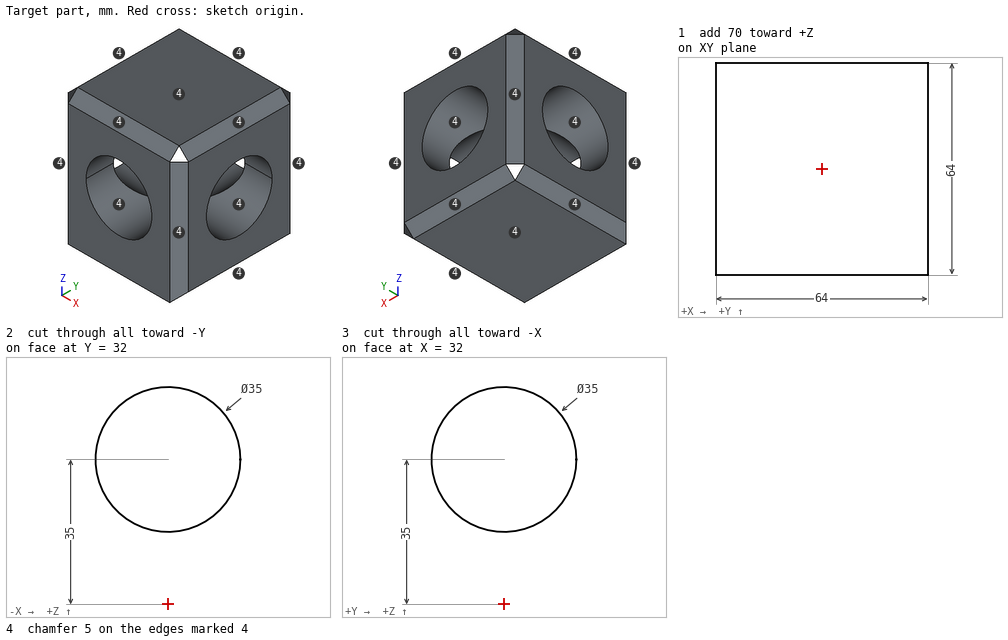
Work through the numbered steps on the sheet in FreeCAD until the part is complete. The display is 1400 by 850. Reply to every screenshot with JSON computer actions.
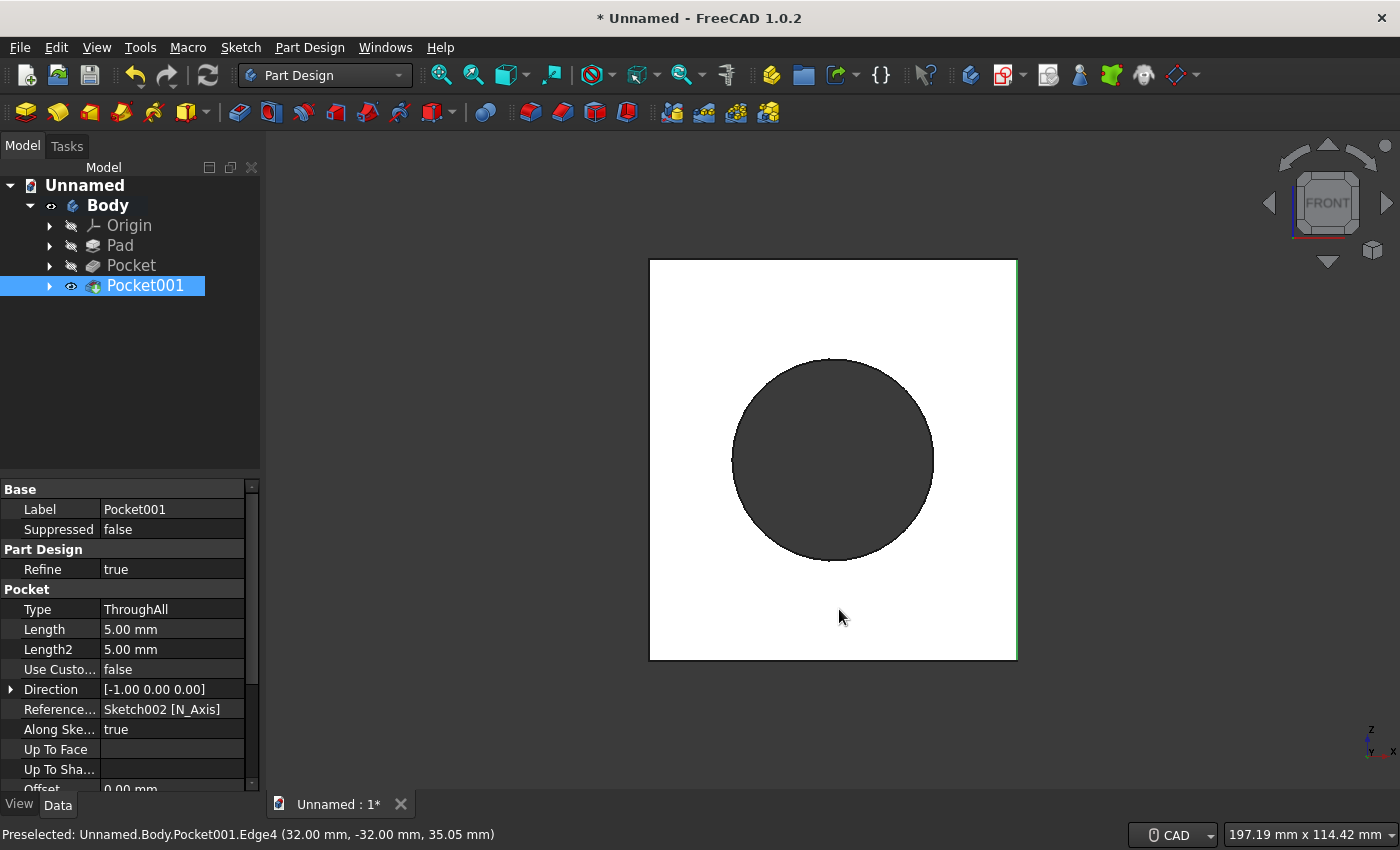
{"action": "left_click", "coordinate": [649, 459], "text": "ctrl"}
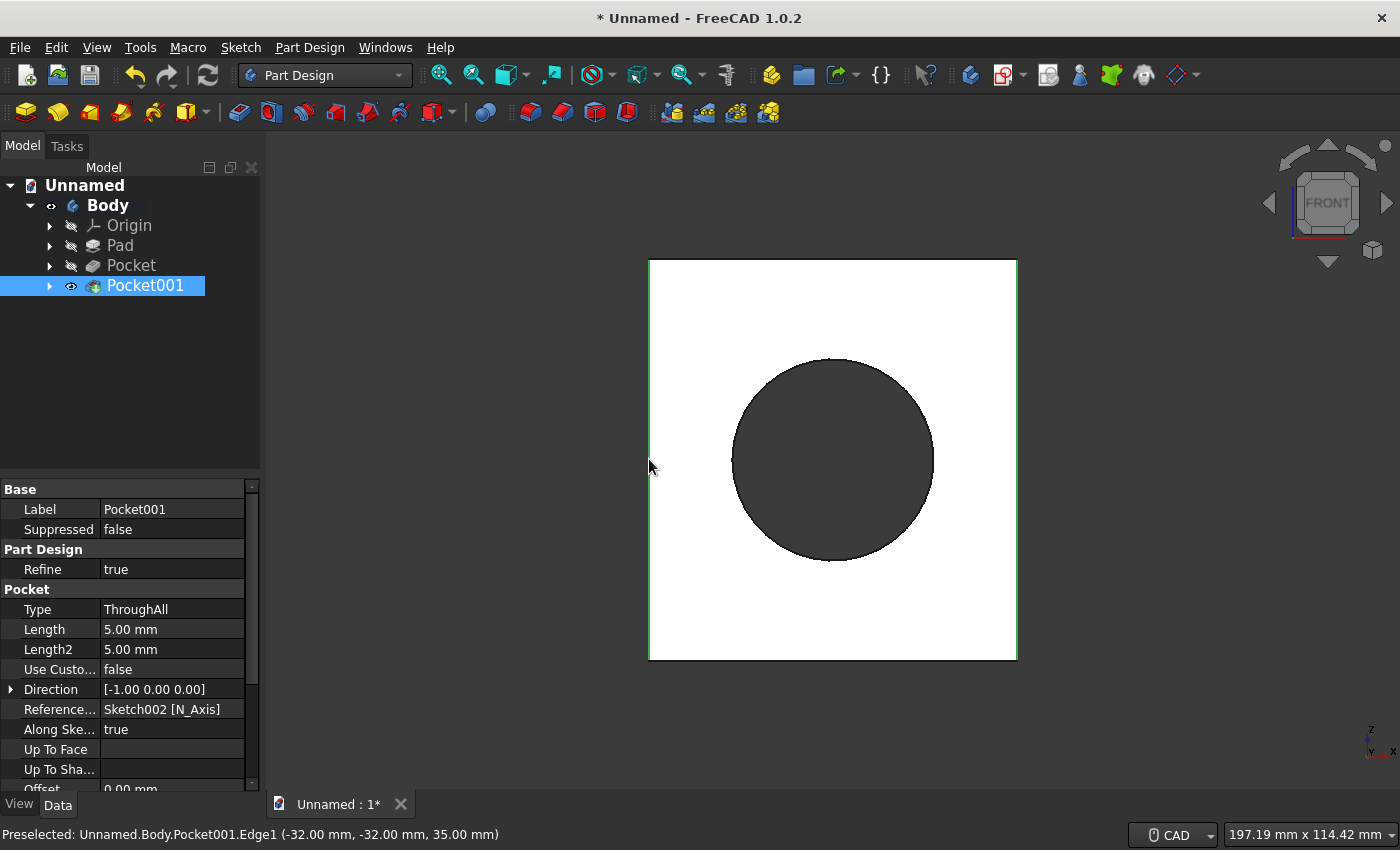
{"action": "key", "text": "3"}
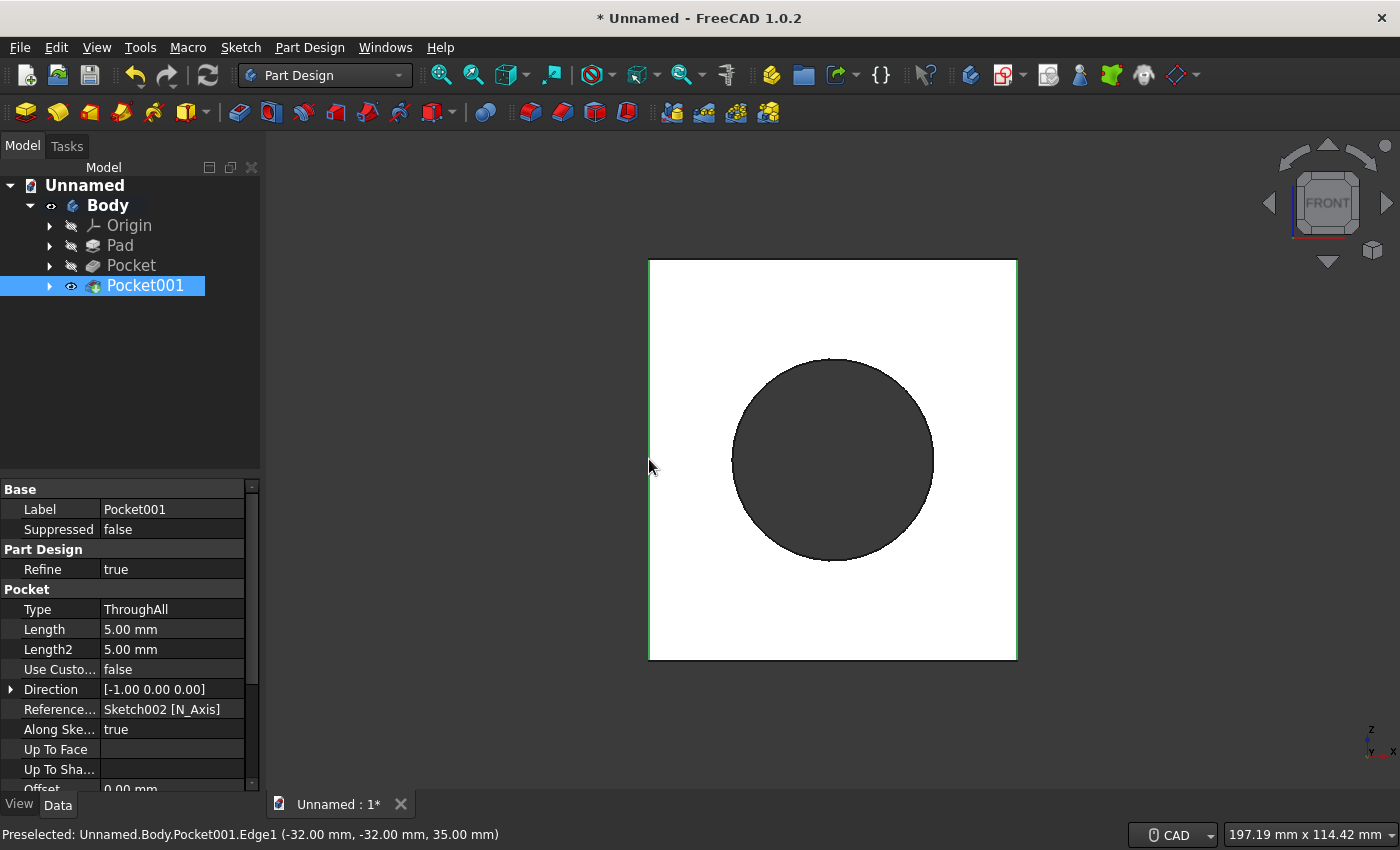
{"action": "left_click", "coordinate": [833, 660], "text": "ctrl"}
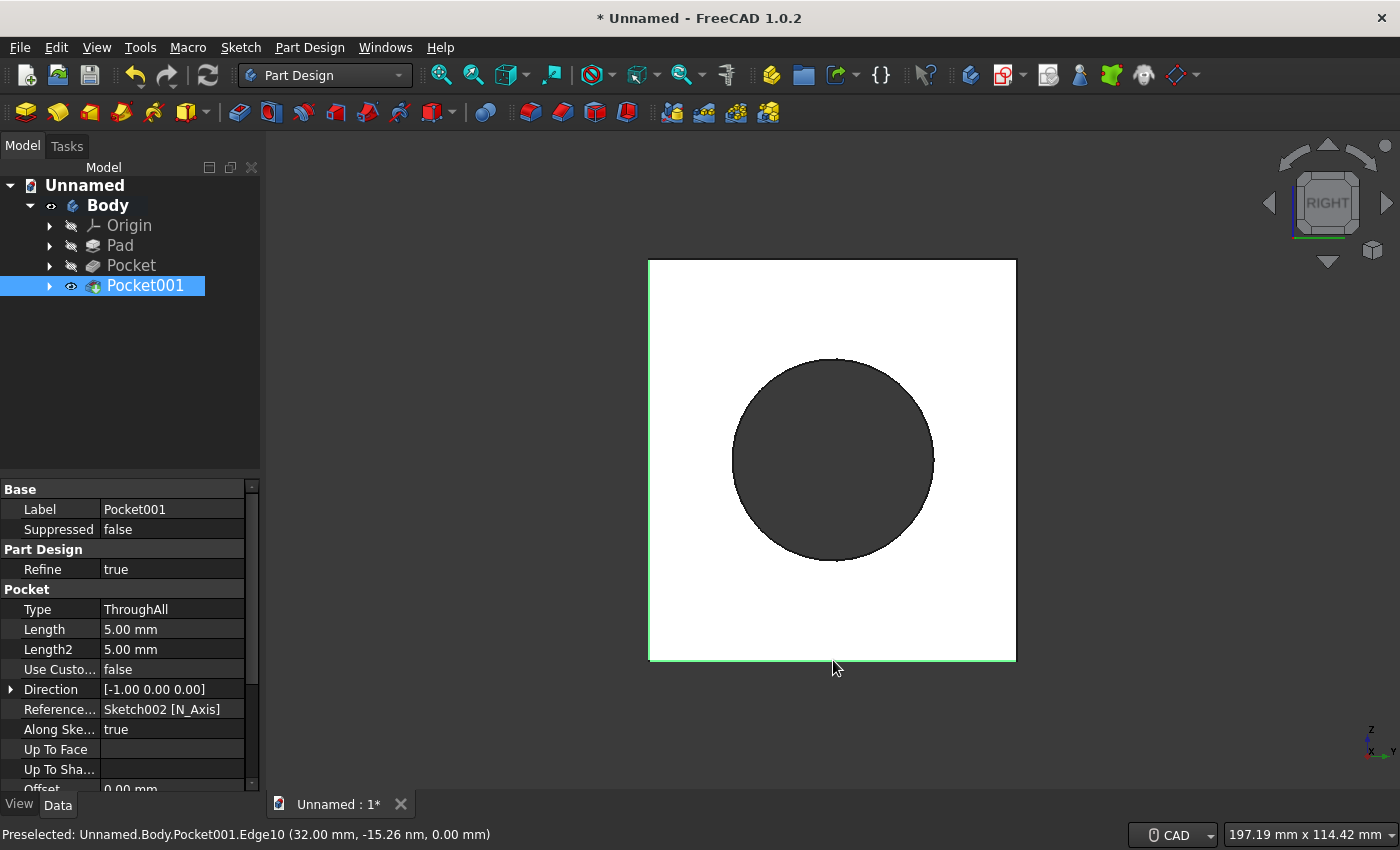
{"action": "left_click", "coordinate": [1017, 459], "text": "ctrl"}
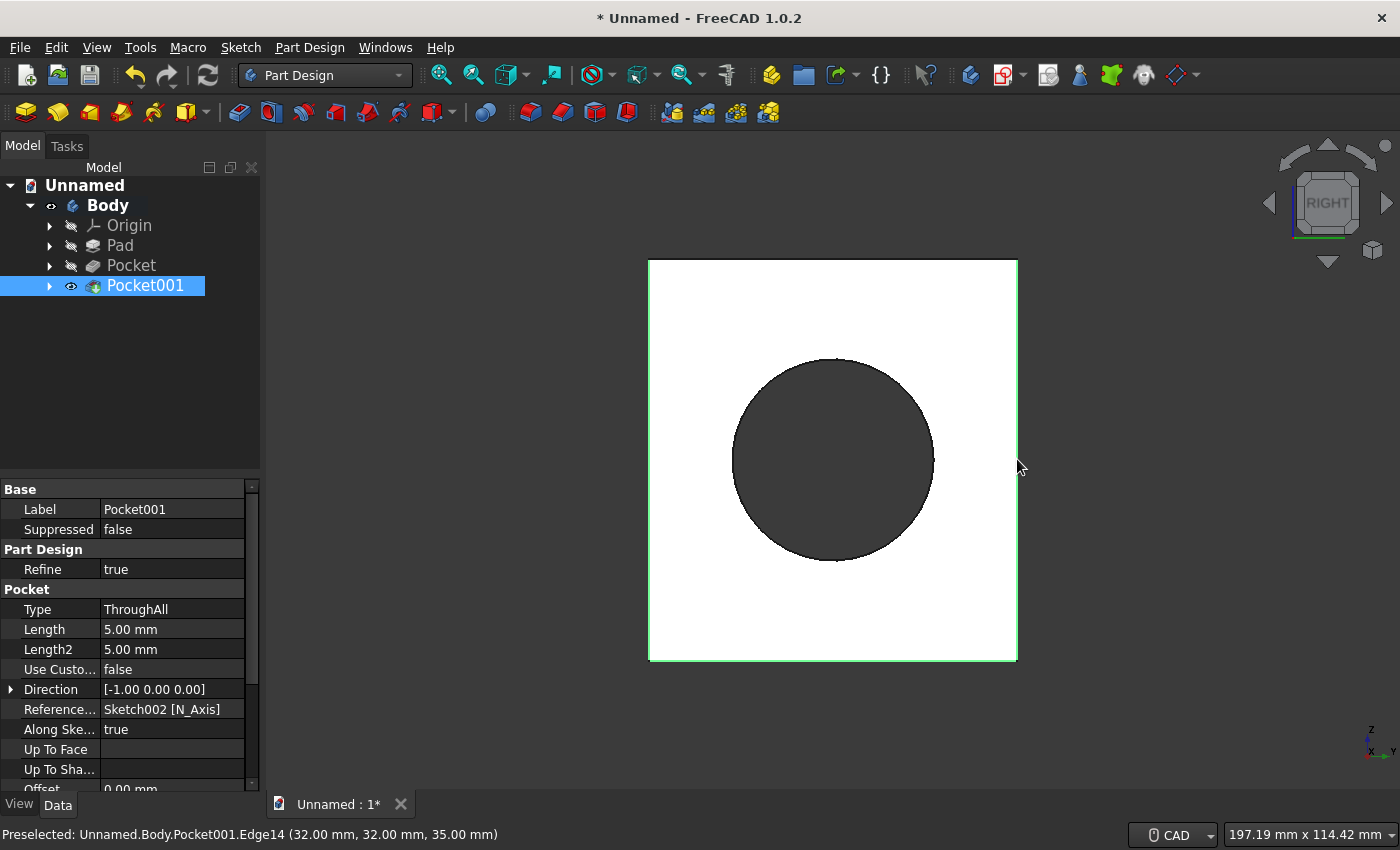
{"action": "key", "text": "5"}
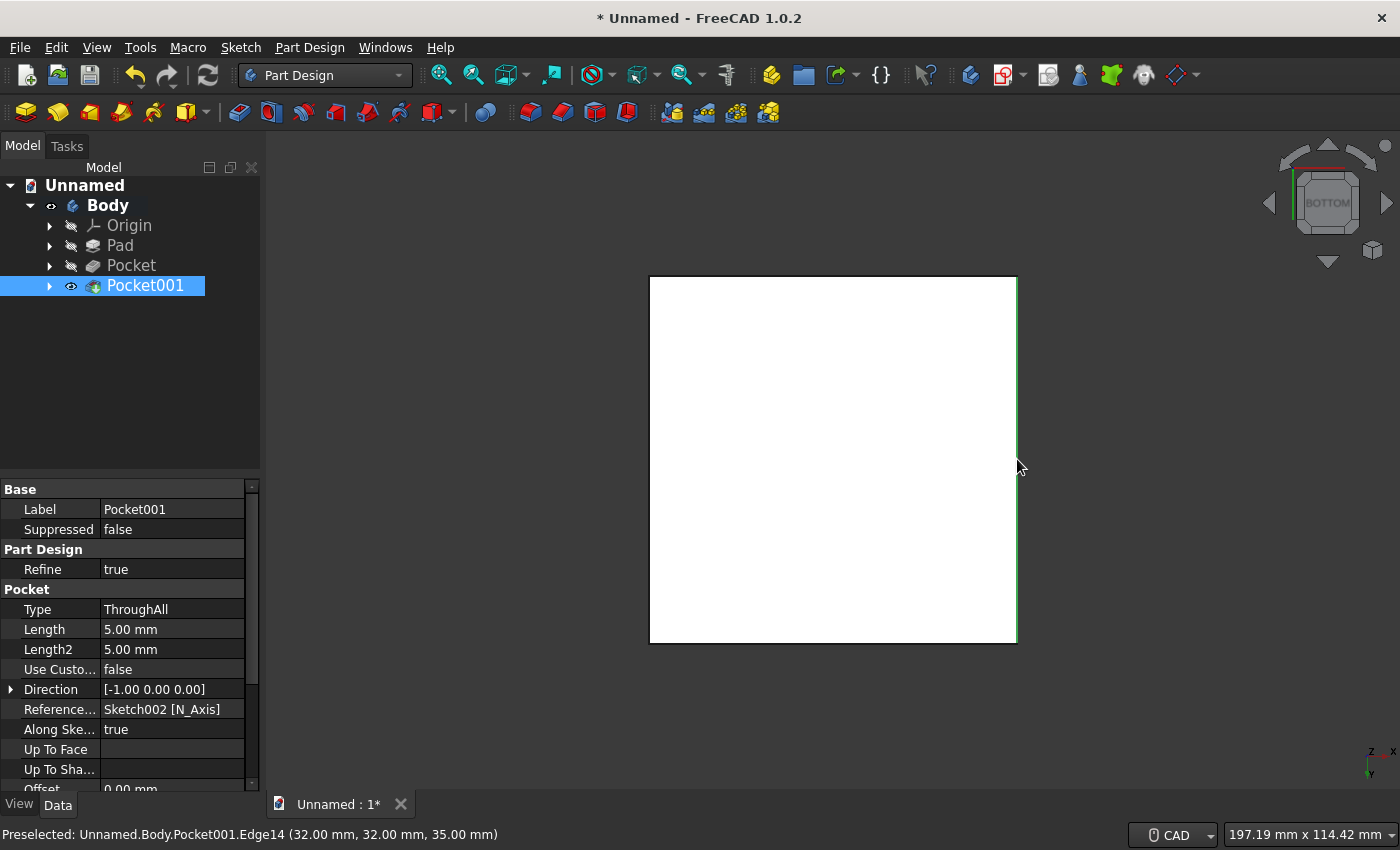
{"action": "left_click", "coordinate": [833, 643], "text": "ctrl"}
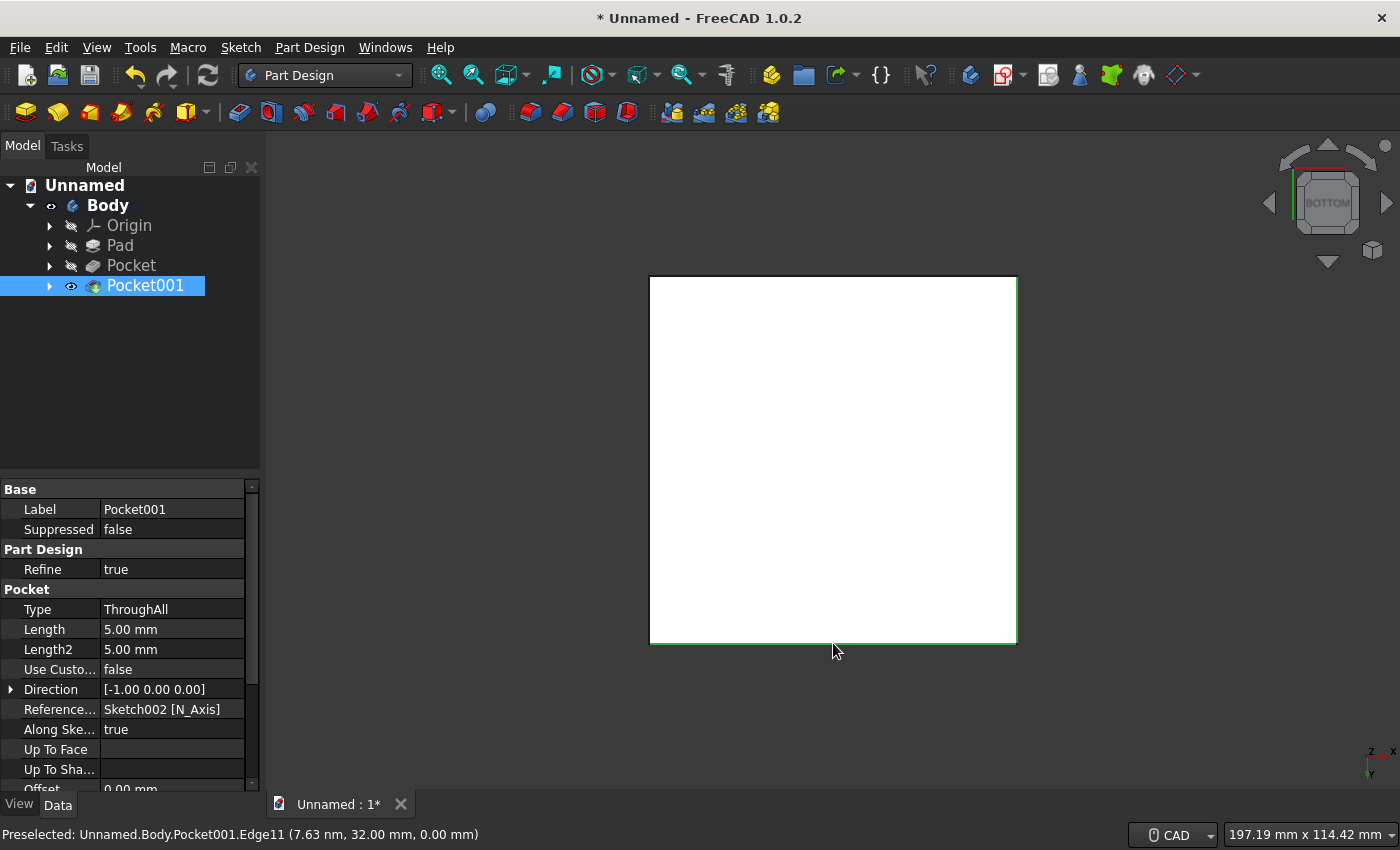
{"action": "left_click", "coordinate": [649, 459], "text": "ctrl"}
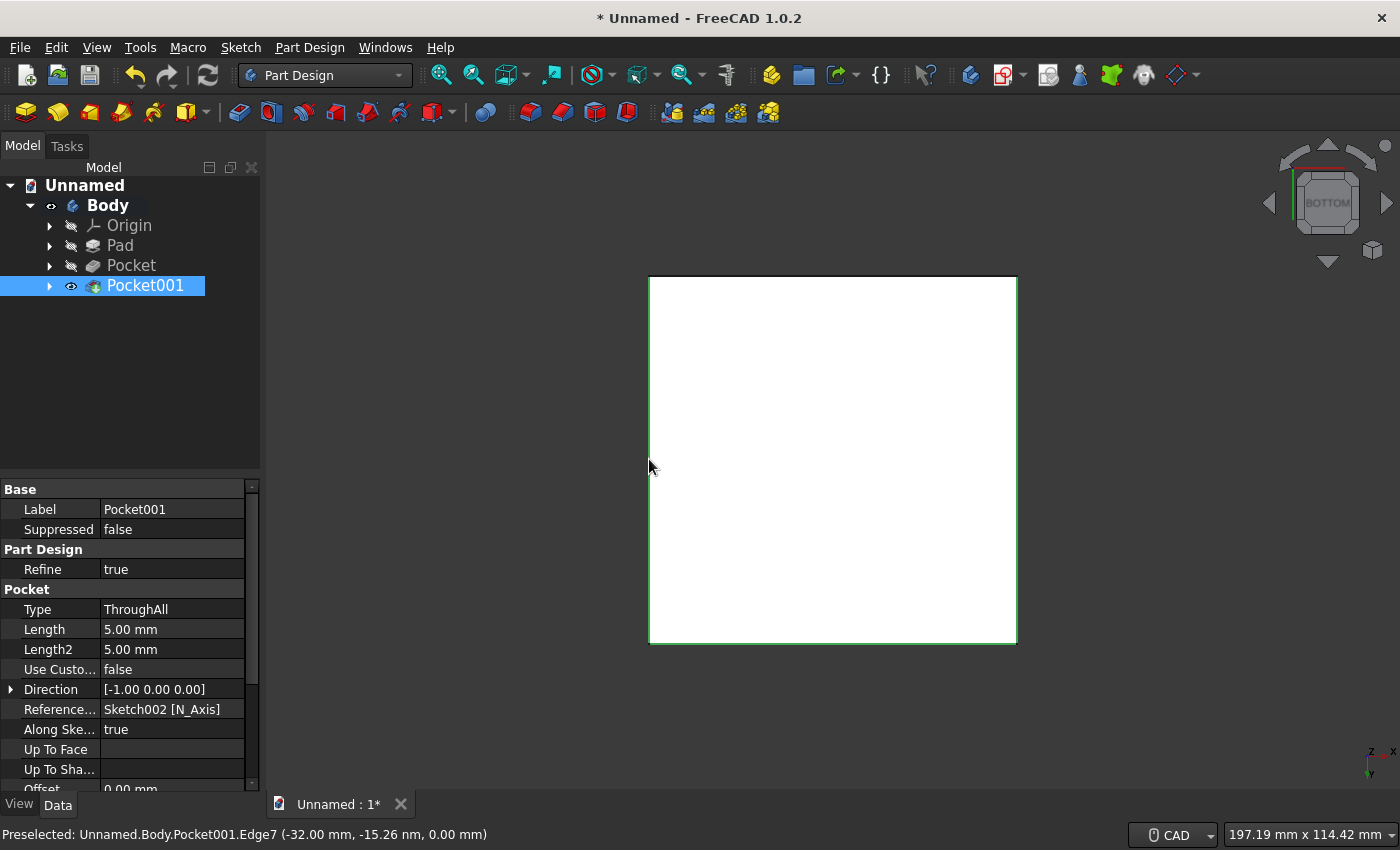
{"action": "key", "text": "4"}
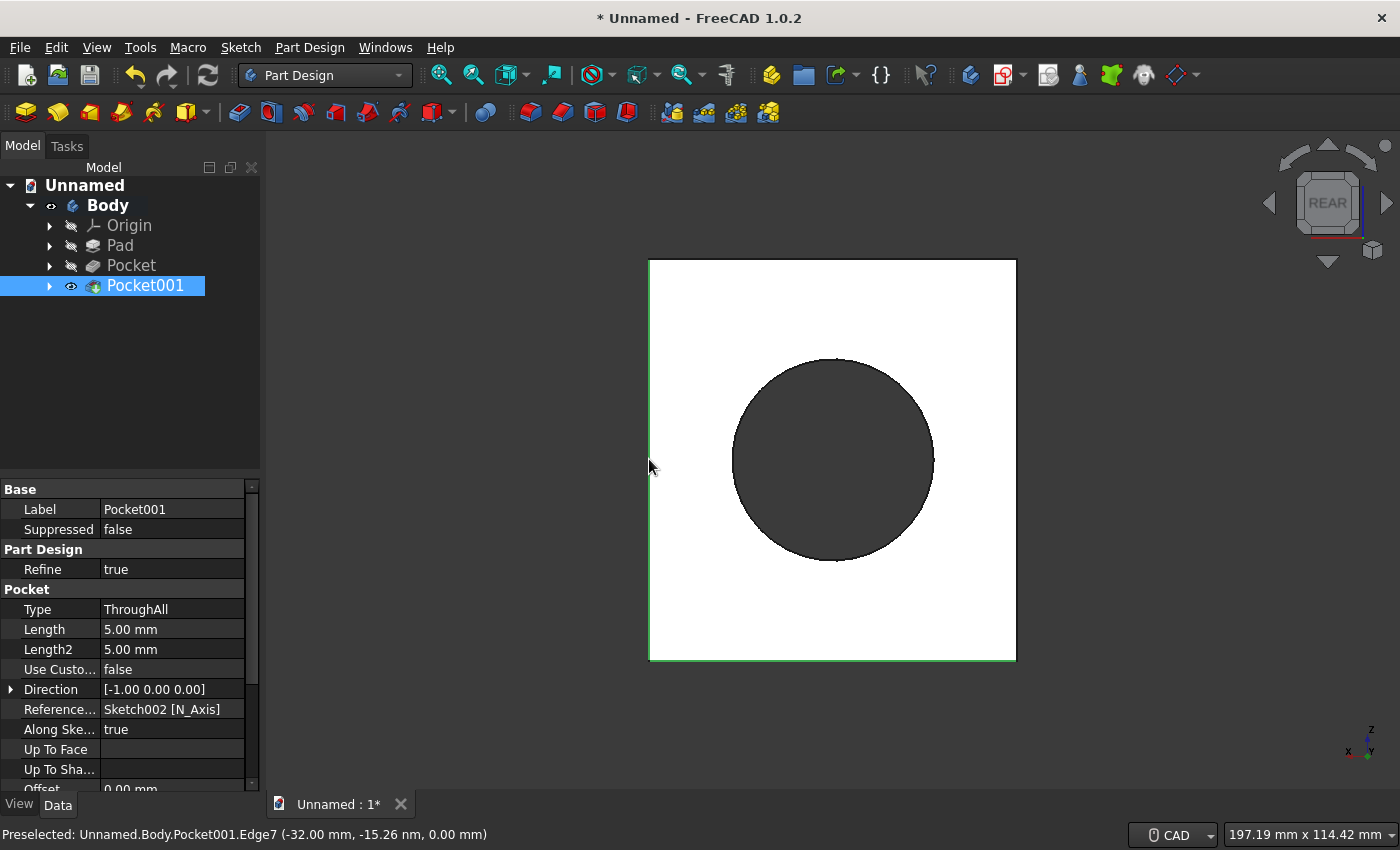
{"action": "left_click", "coordinate": [1017, 459], "text": "ctrl"}